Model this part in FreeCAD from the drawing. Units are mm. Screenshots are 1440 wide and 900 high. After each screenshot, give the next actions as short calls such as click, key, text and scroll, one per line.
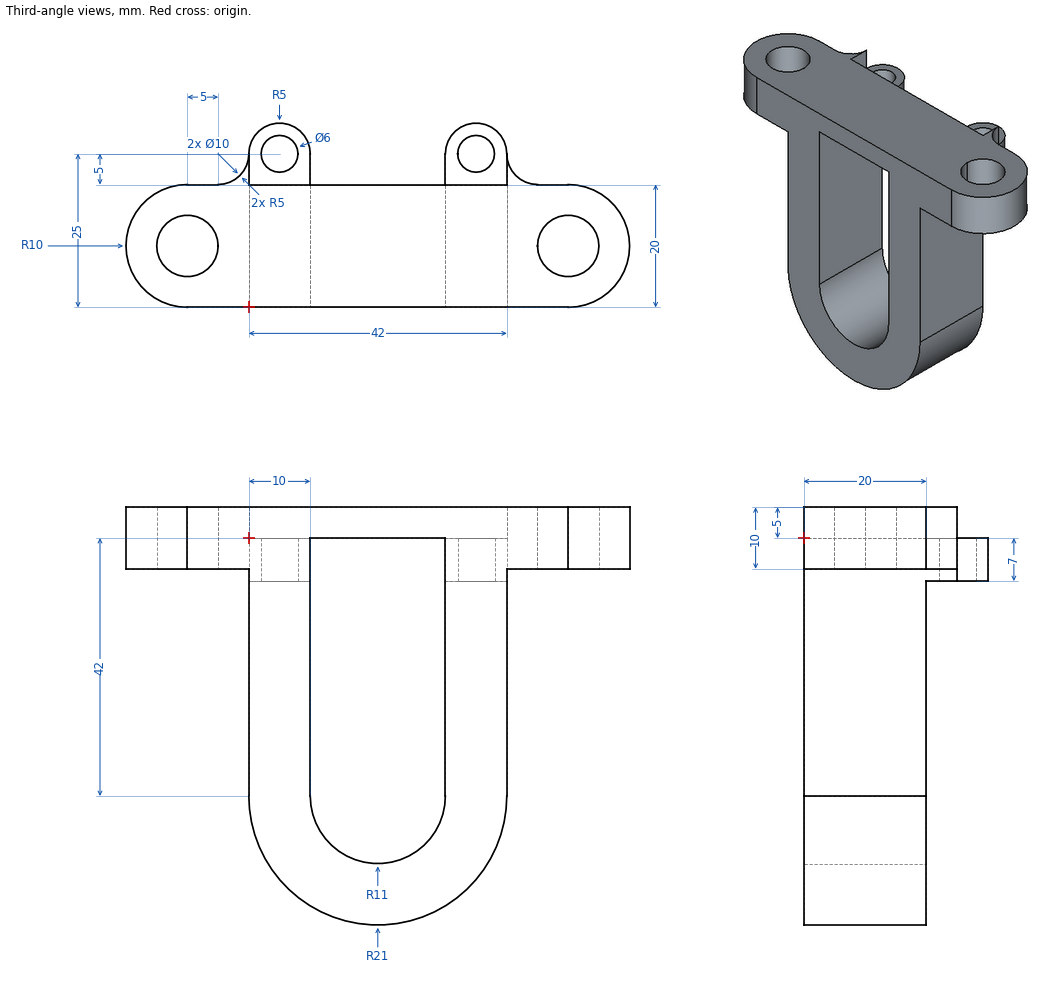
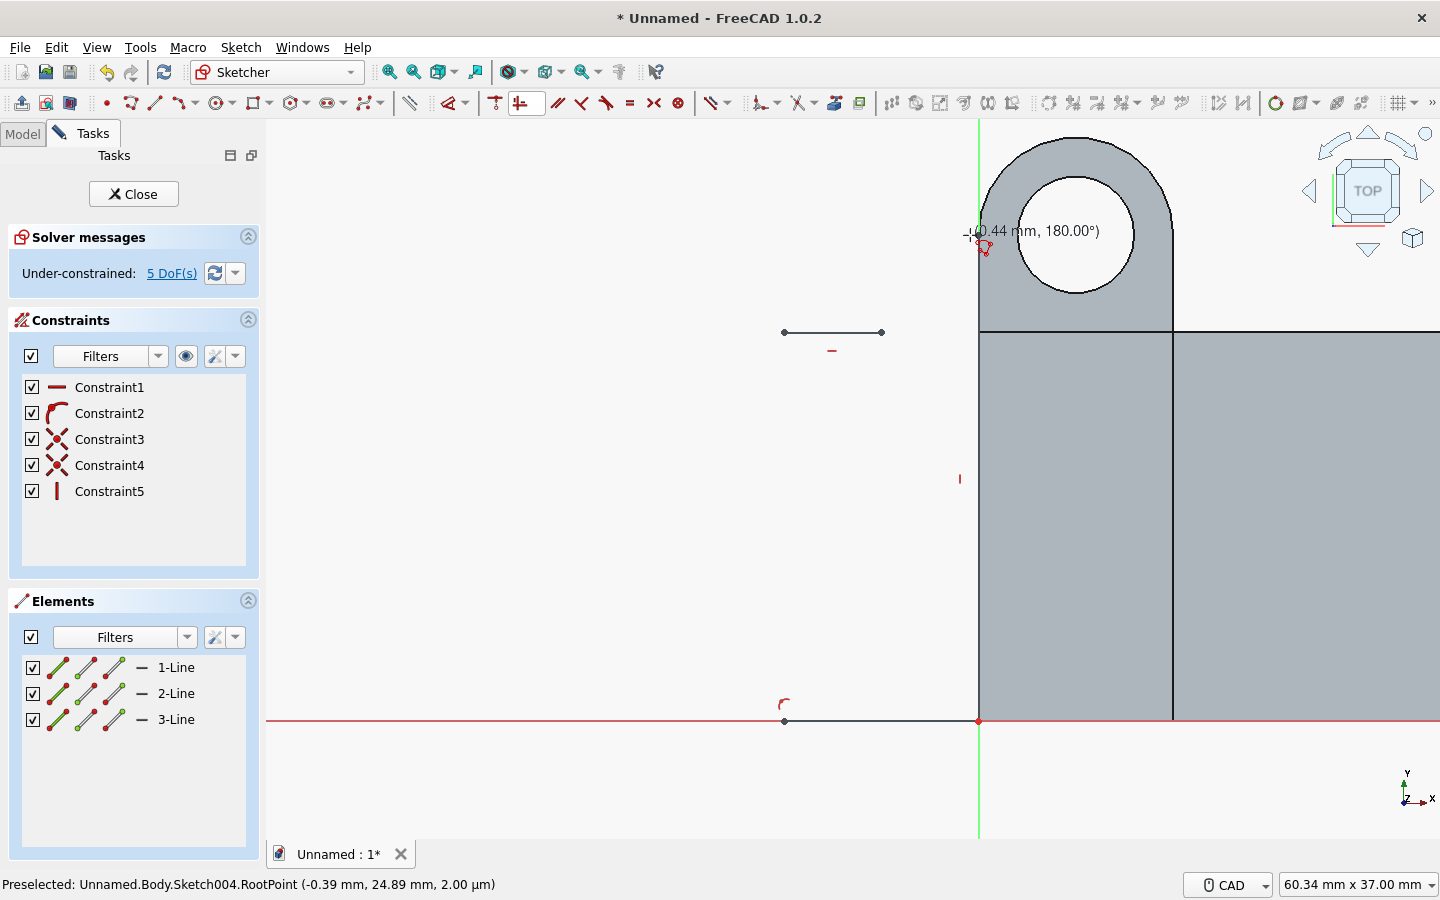
click(180, 104)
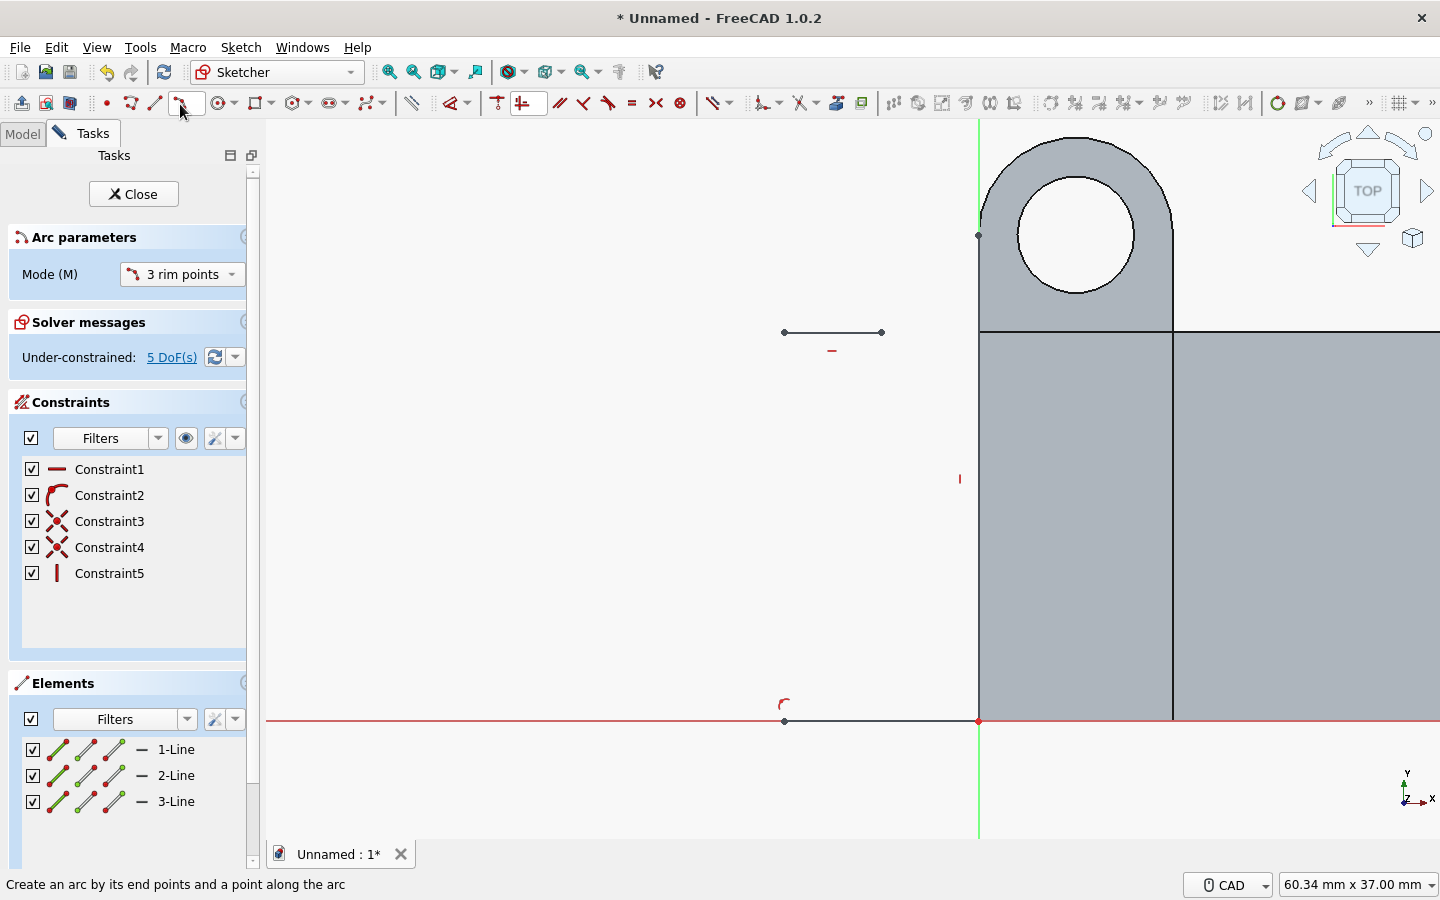
click(784, 333)
click(784, 721)
click(589, 527)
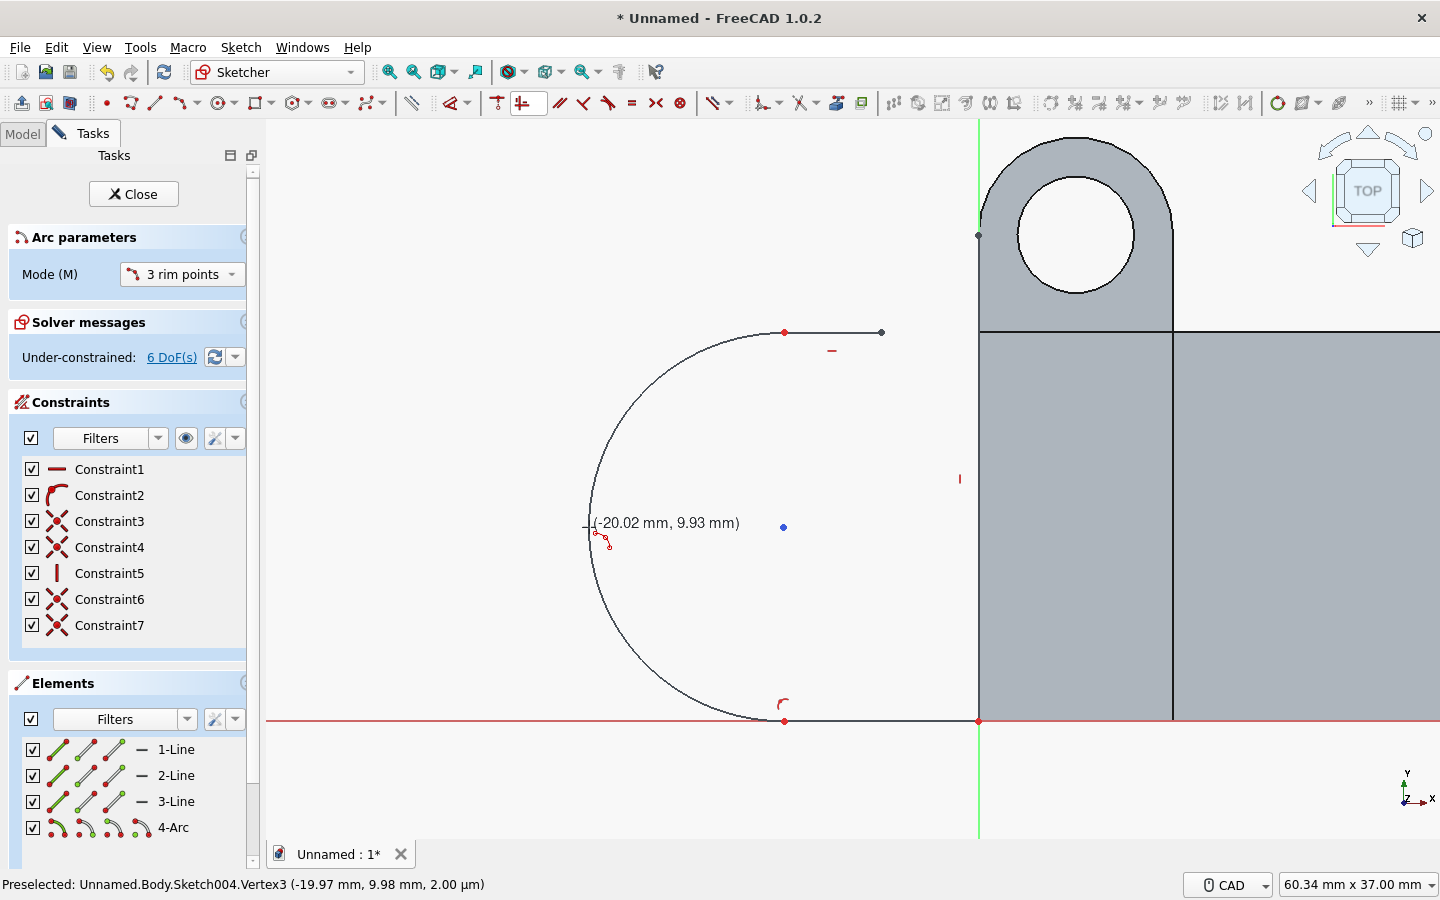
click(979, 236)
click(881, 333)
click(950, 304)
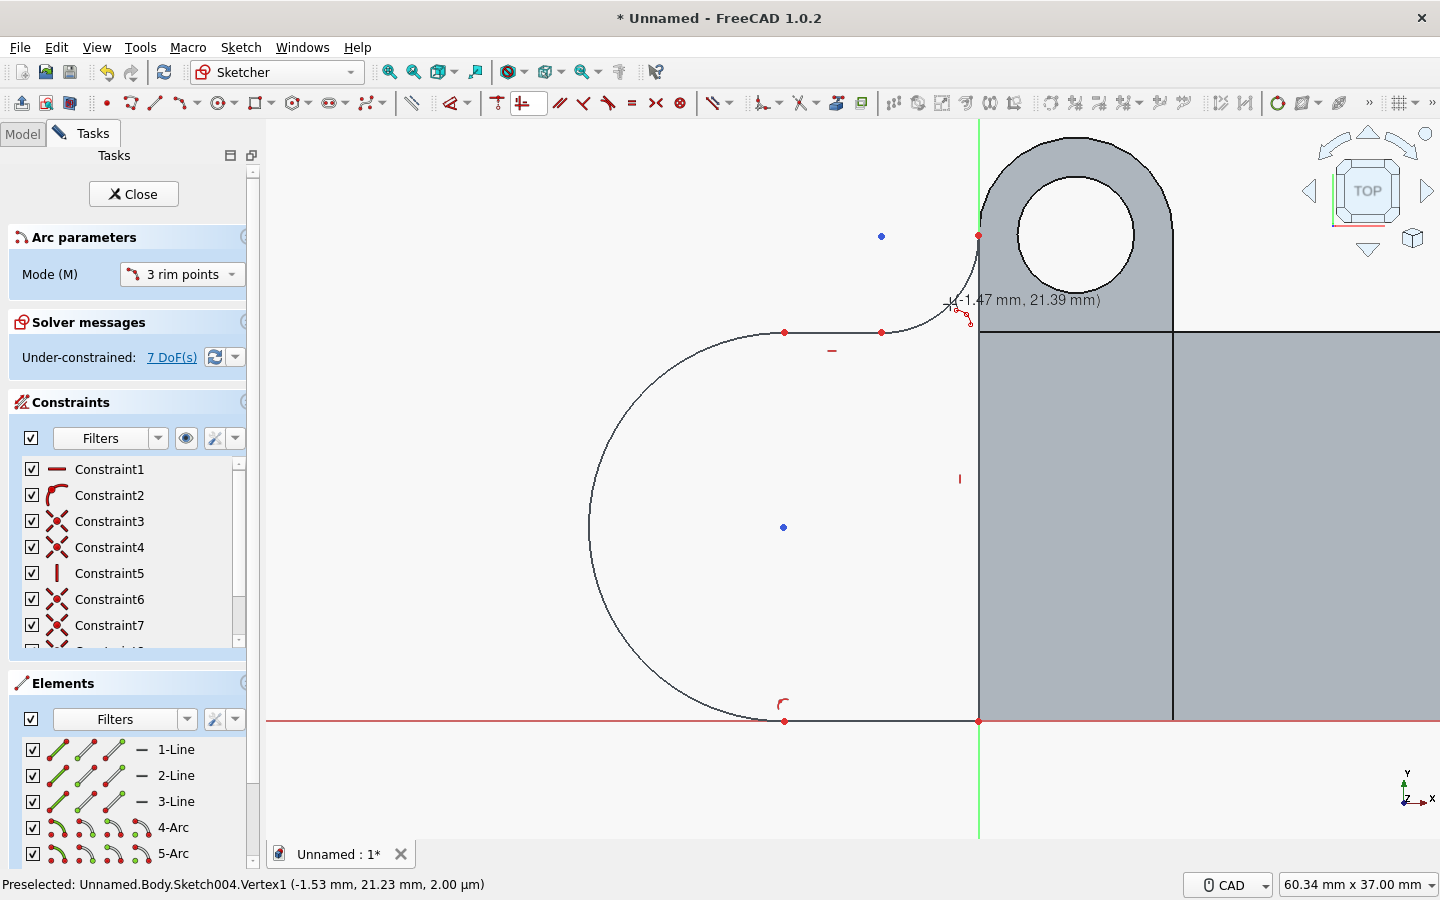
click(218, 104)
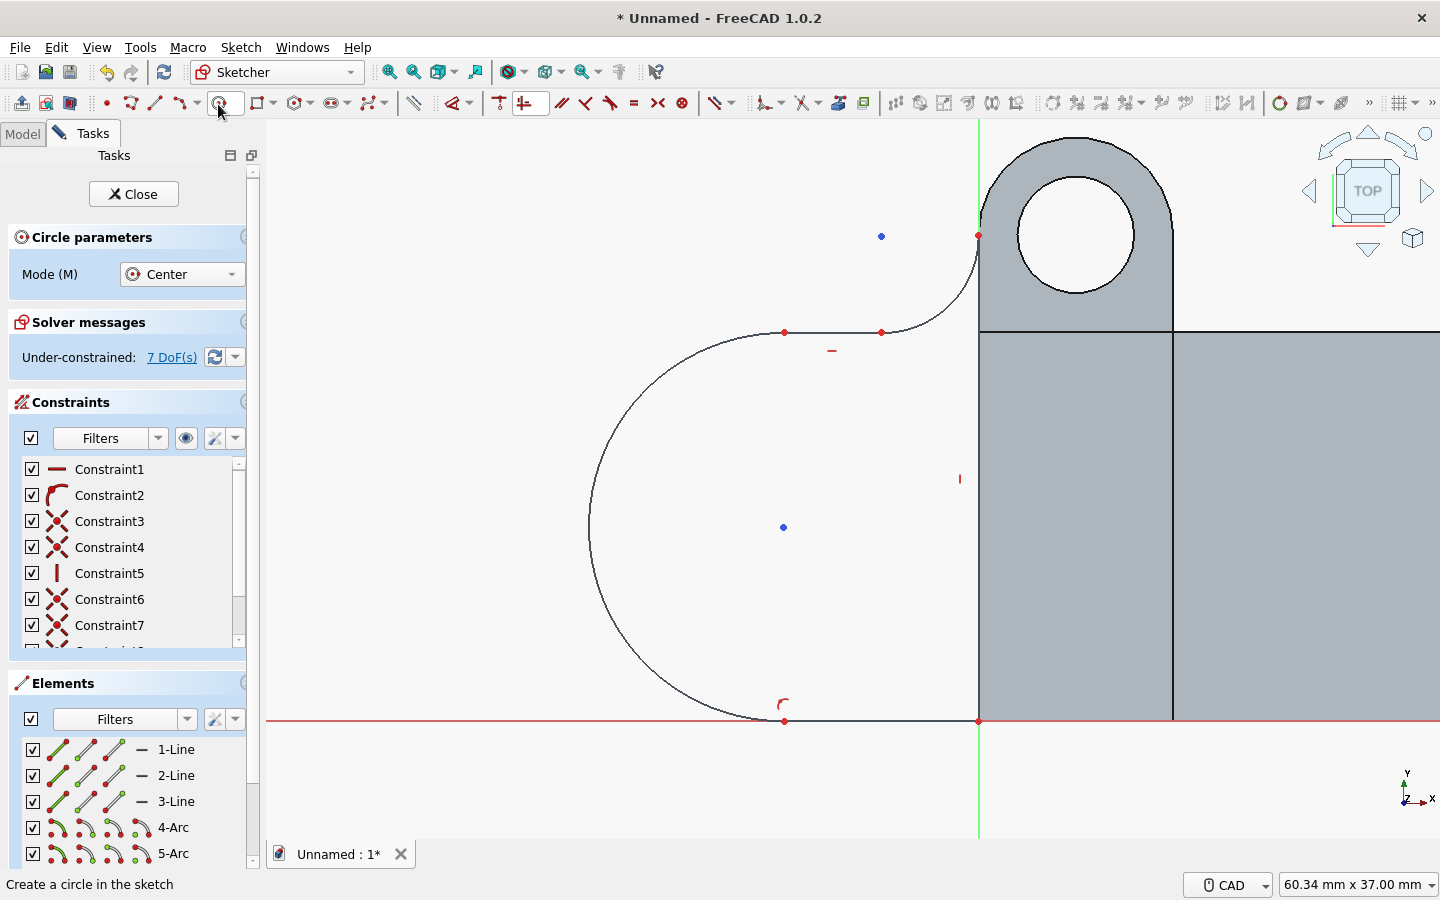
click(784, 527)
click(853, 458)
key(Escape)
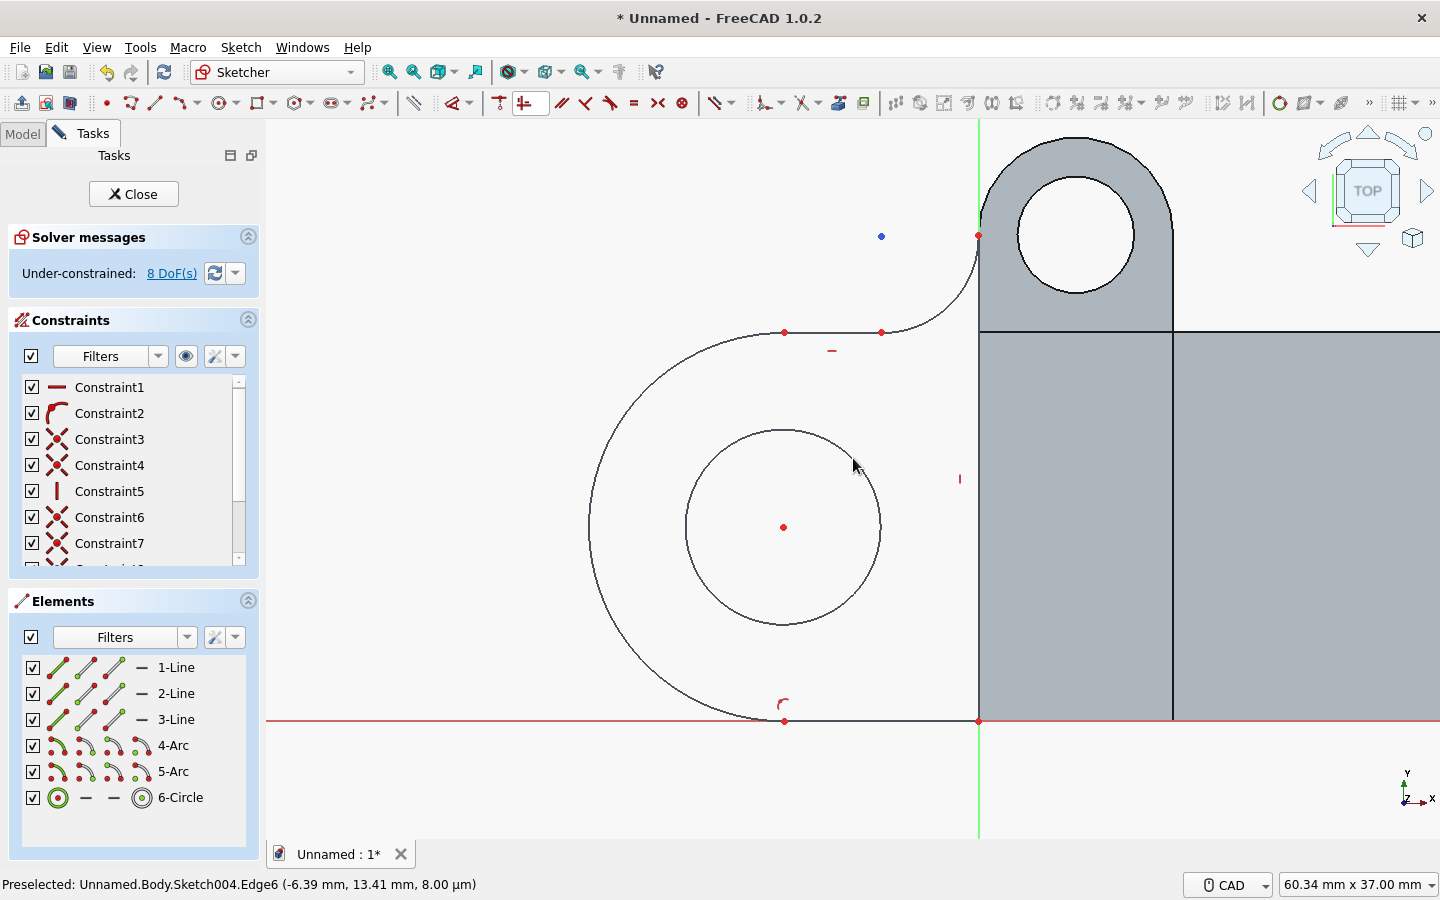
click(852, 333)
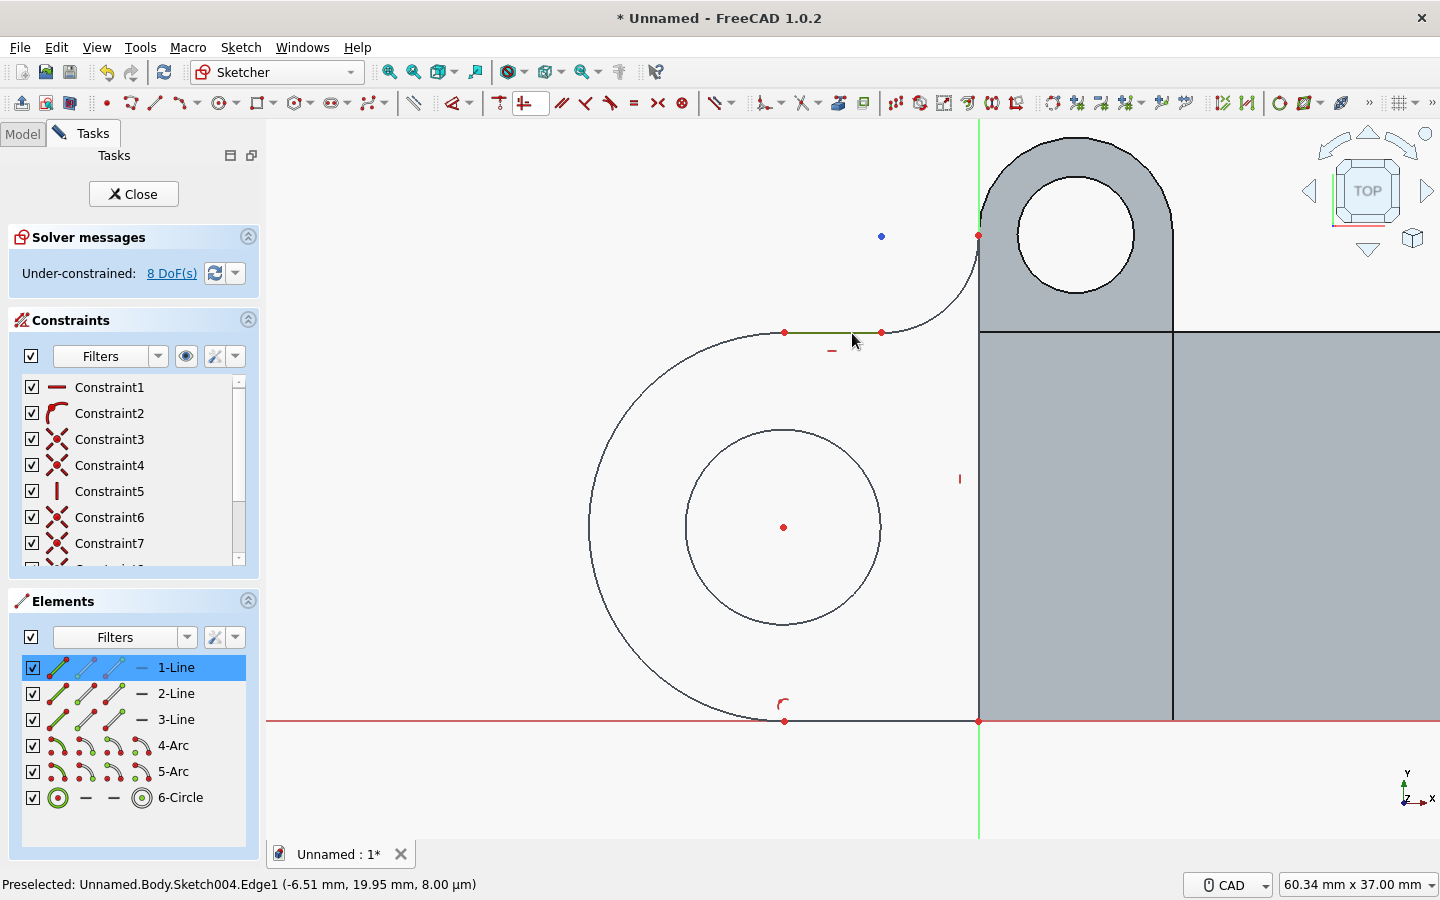
click(626, 413)